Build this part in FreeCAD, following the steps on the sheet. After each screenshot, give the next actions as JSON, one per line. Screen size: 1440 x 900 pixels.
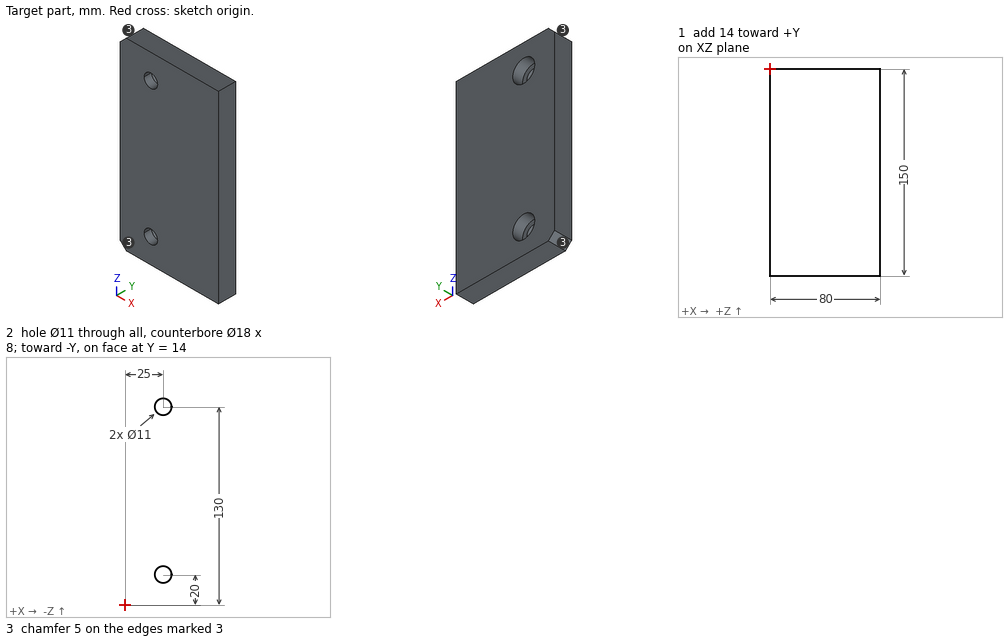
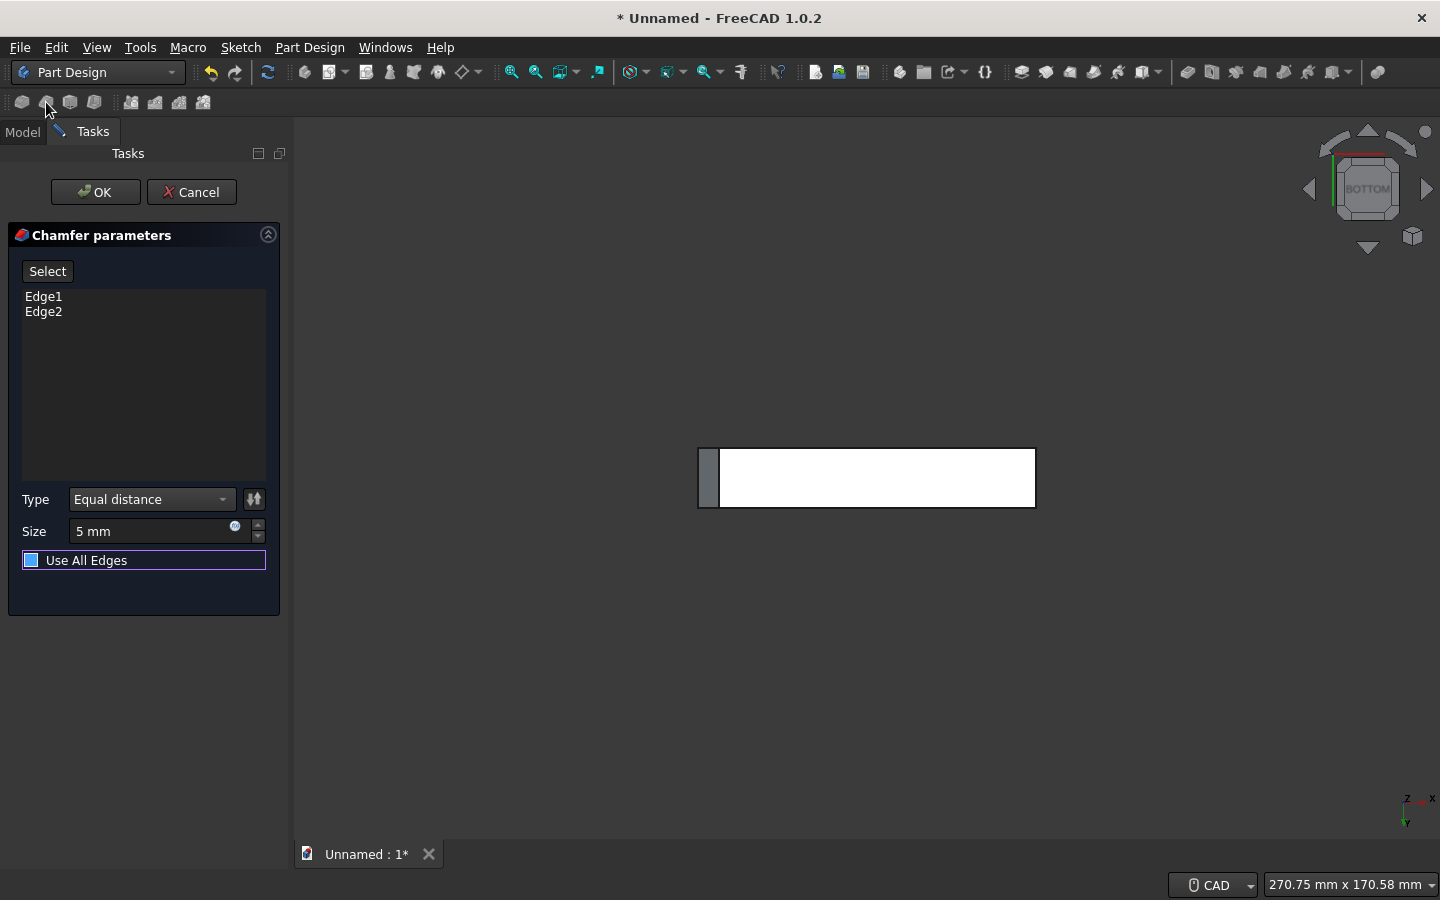
{"action": "left_click", "coordinate": [96, 192]}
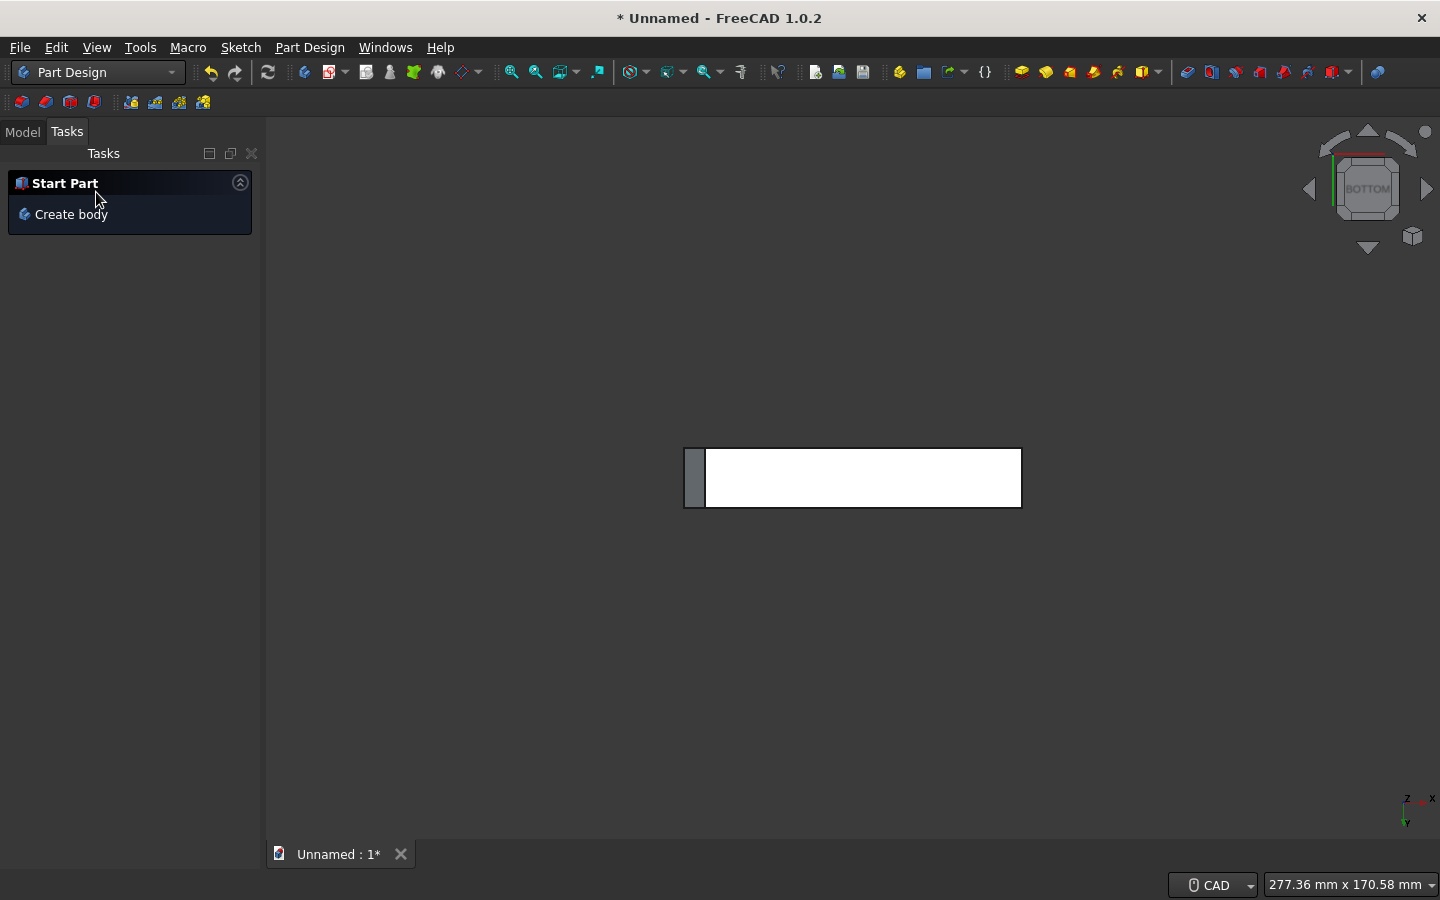
{"action": "key", "text": "0"}